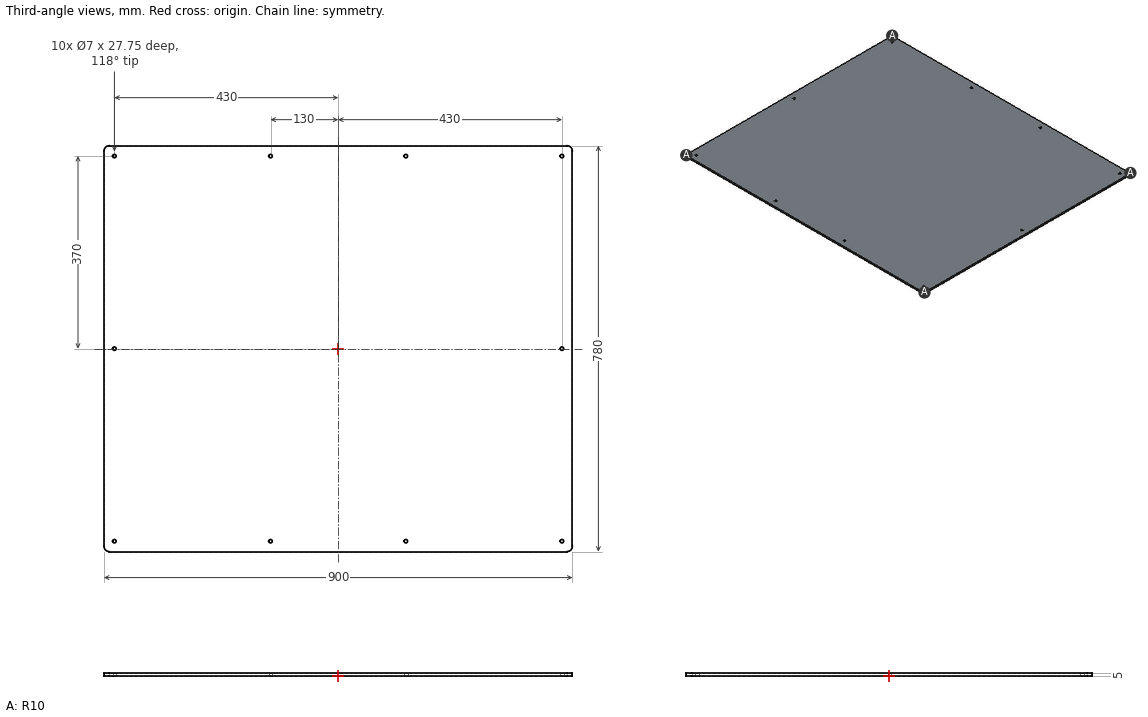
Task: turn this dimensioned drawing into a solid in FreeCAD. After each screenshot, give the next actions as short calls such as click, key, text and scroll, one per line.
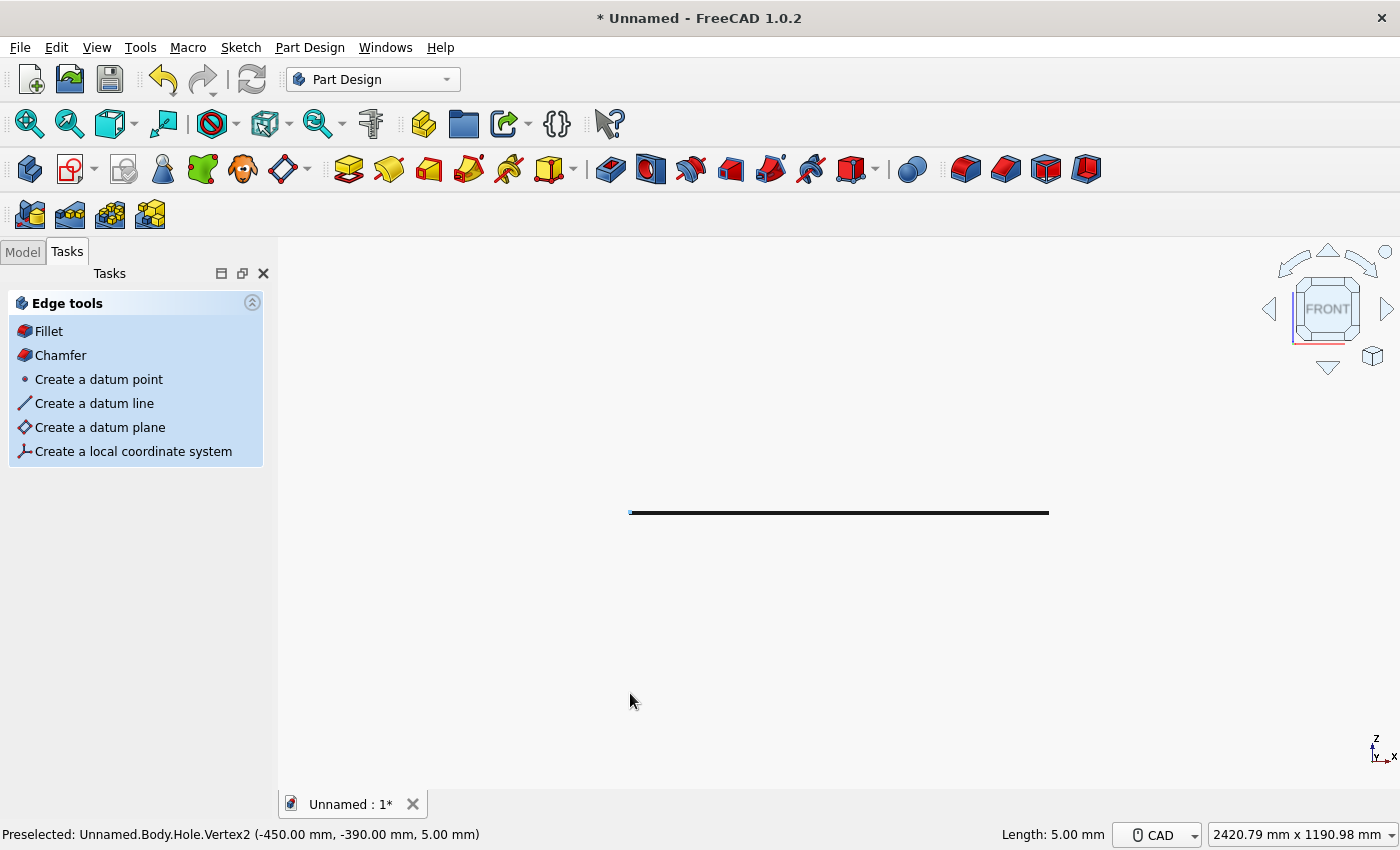
scroll(630, 512, up, 15)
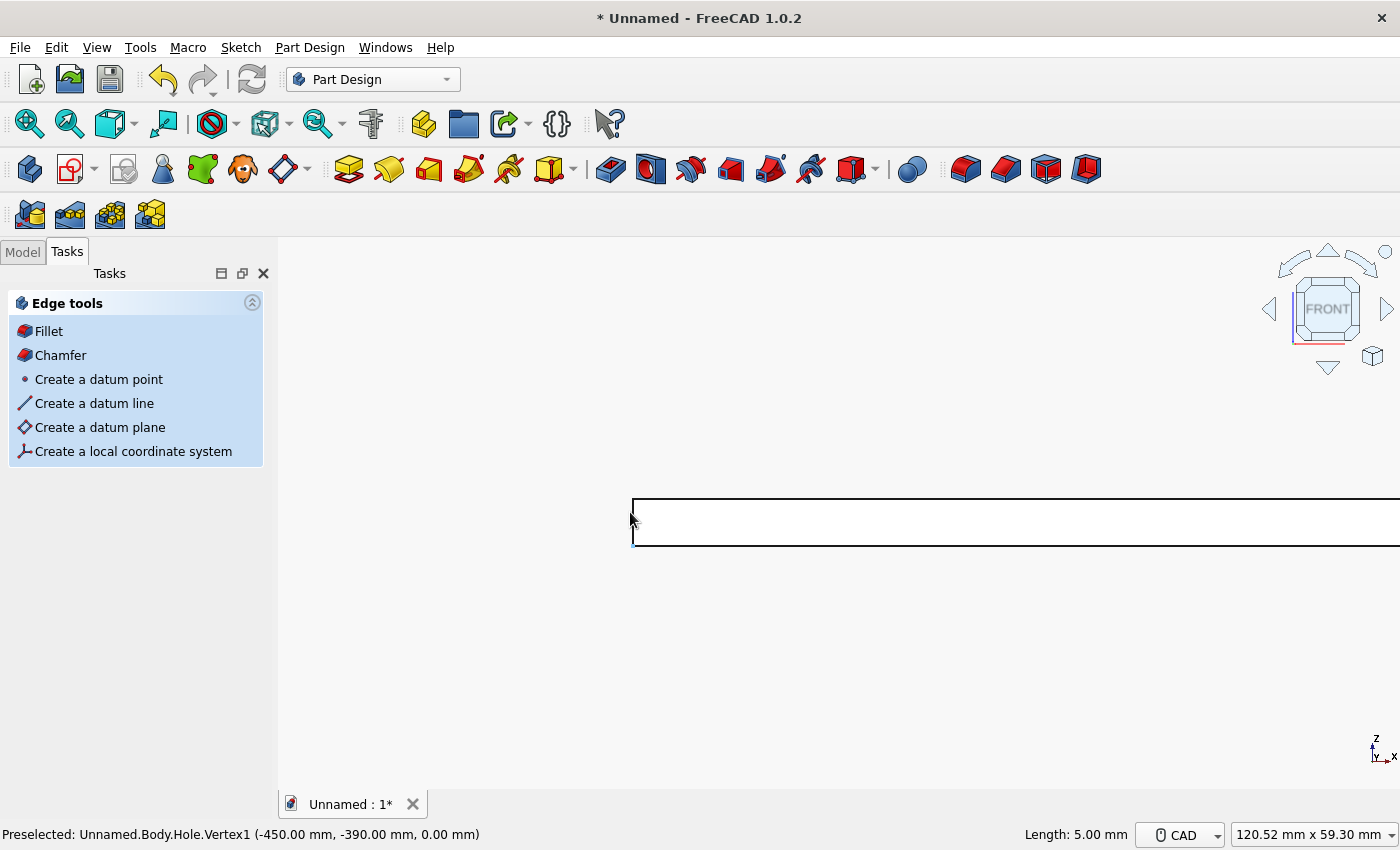
click(633, 522, ctrl)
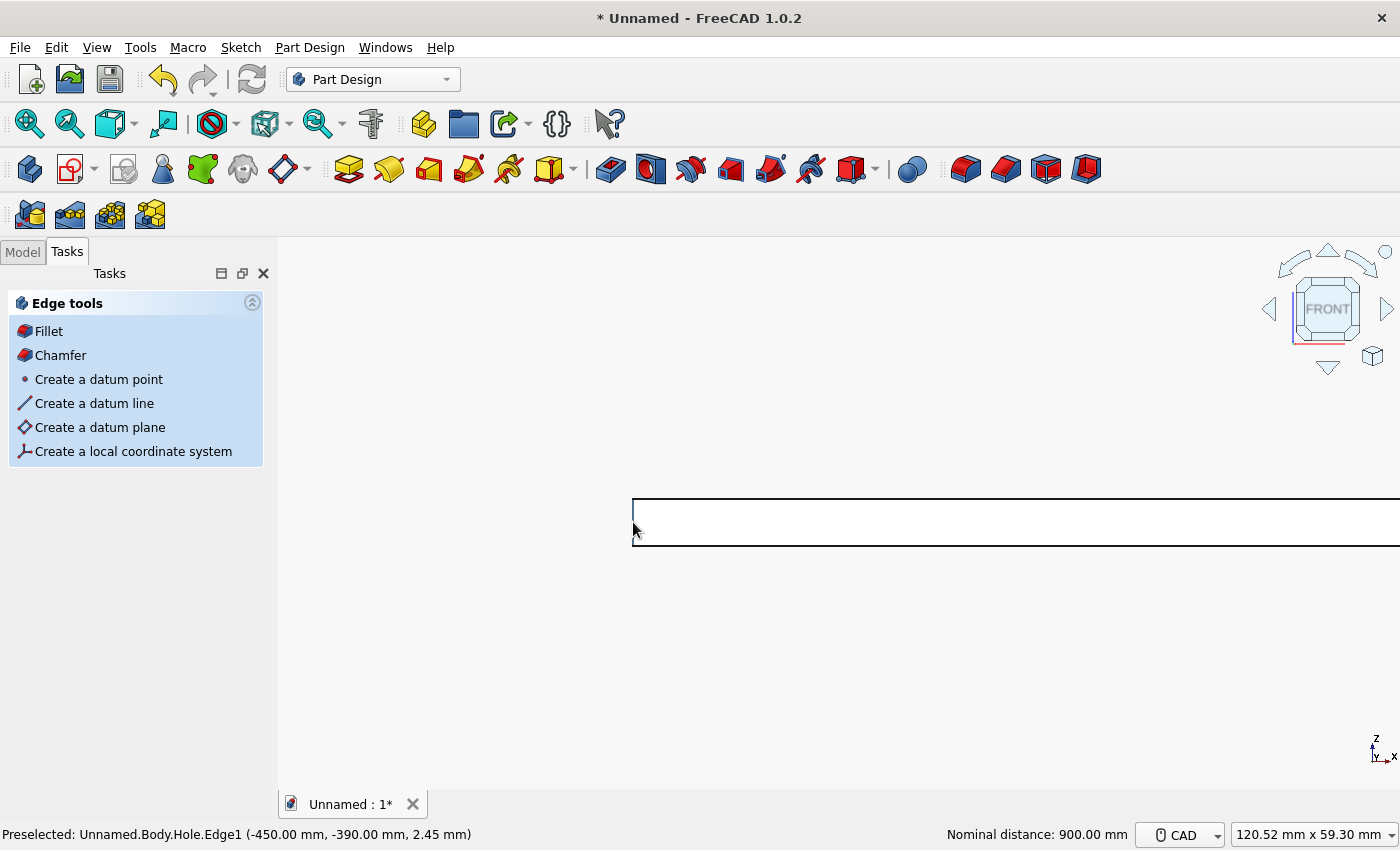
click(30, 124)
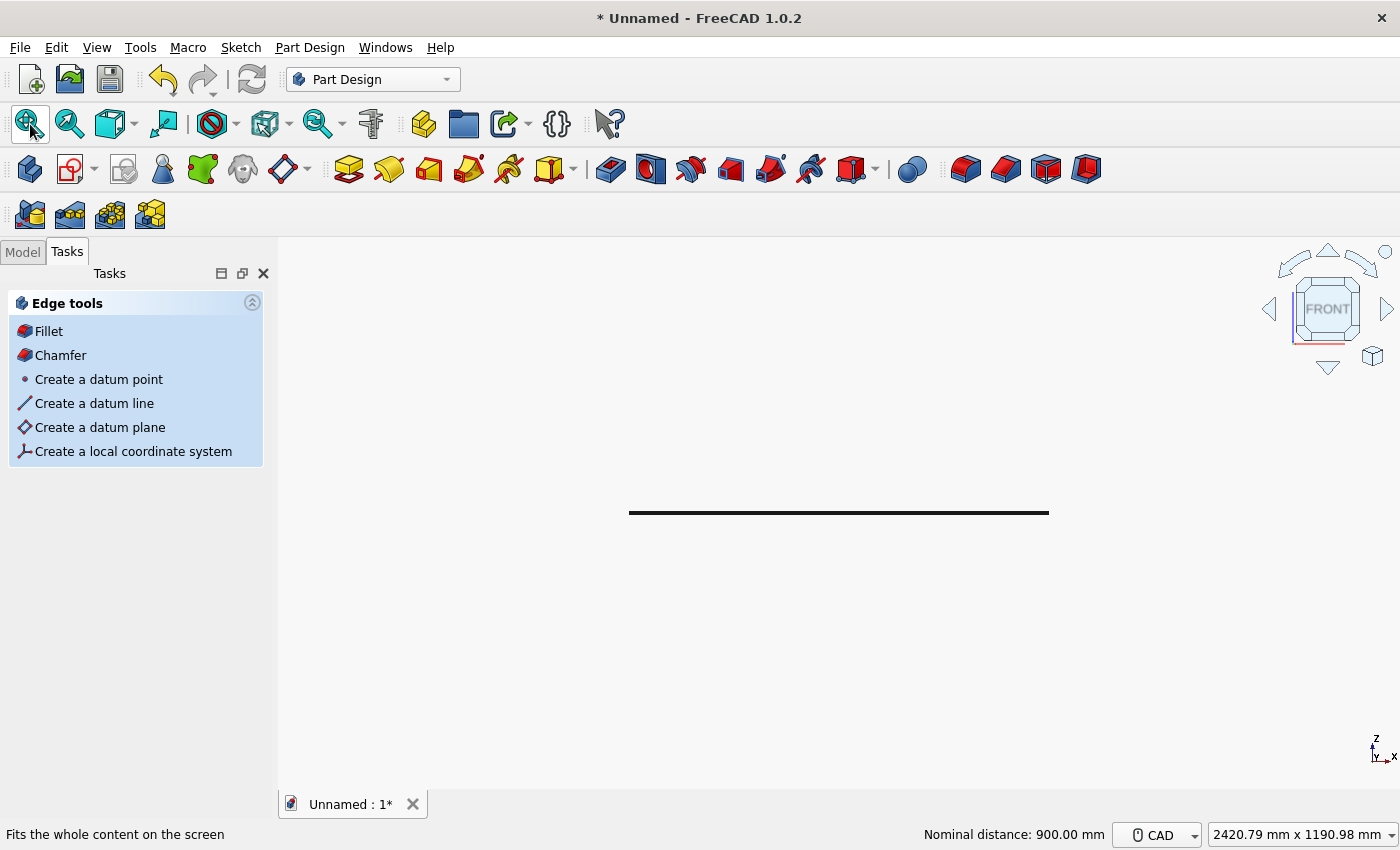
key(3)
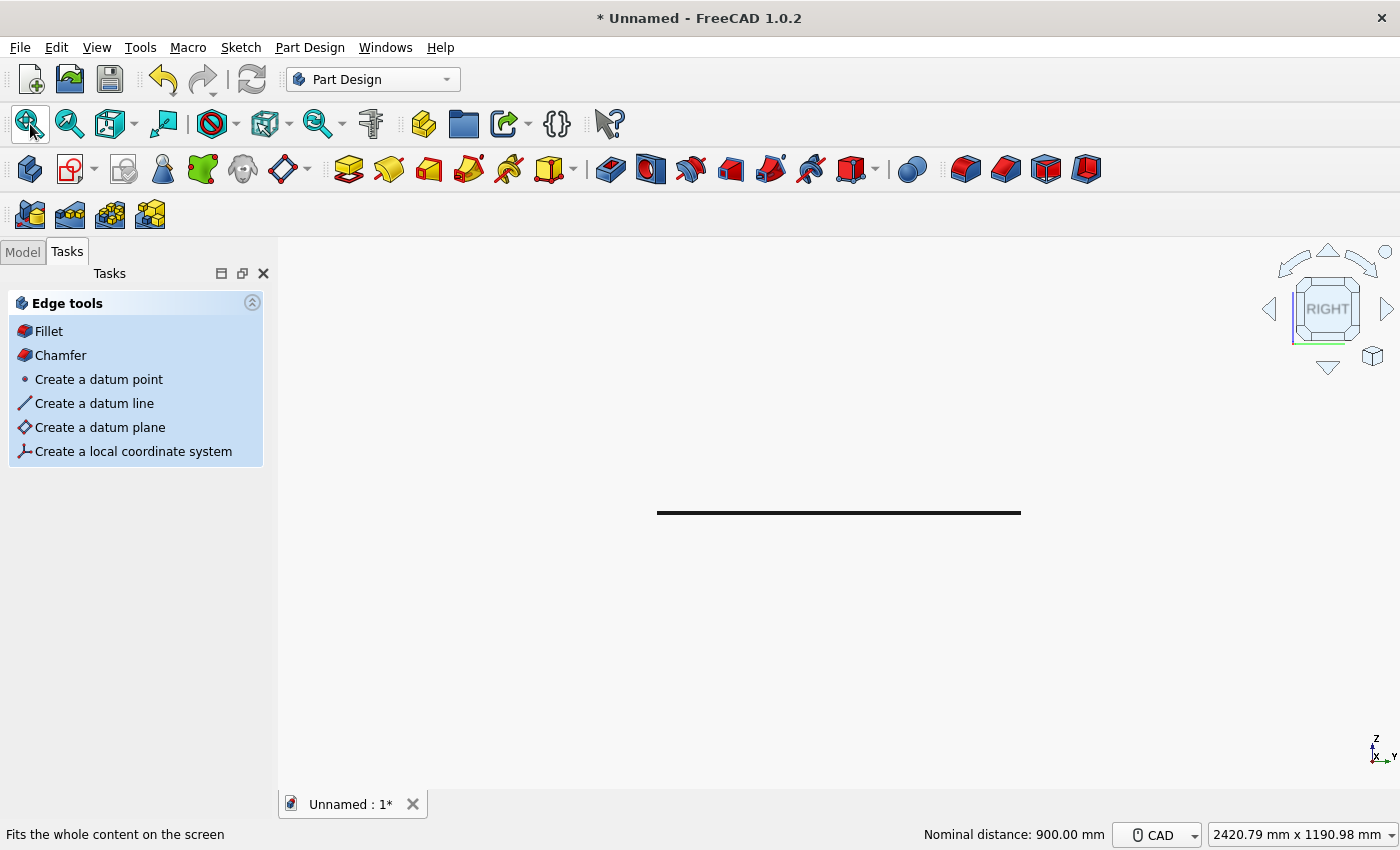
click(30, 124)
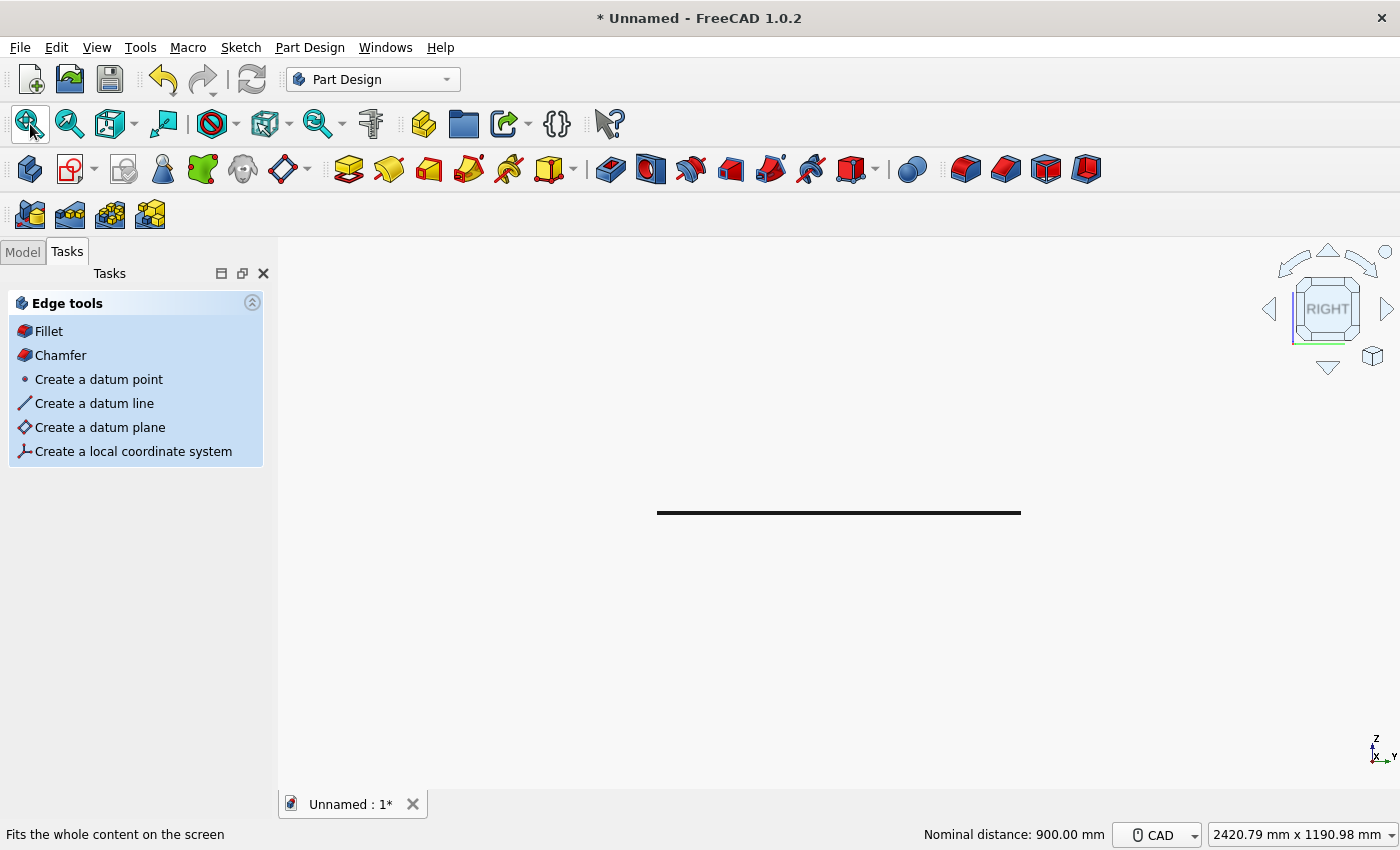
scroll(1020, 512, up, 15)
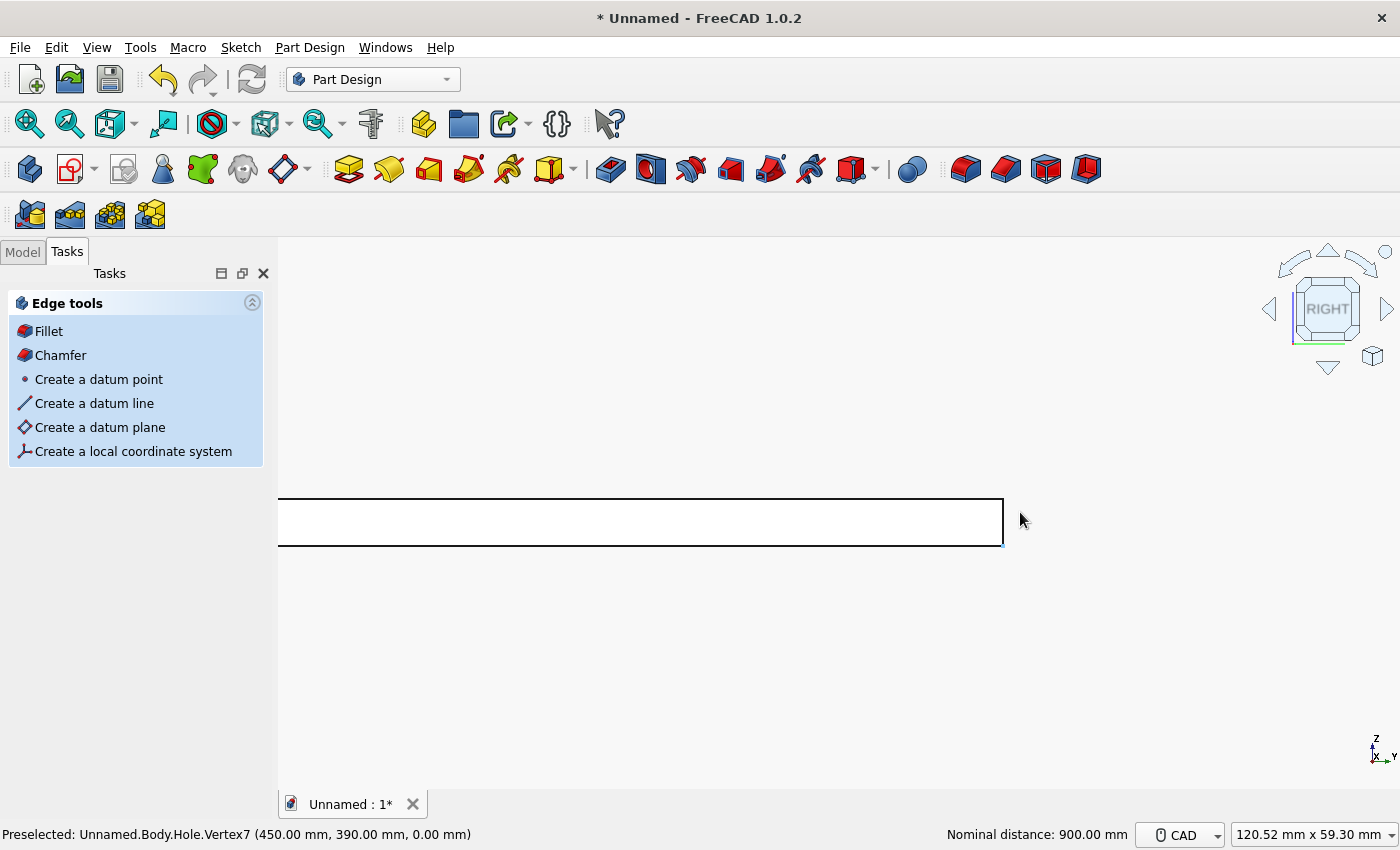
click(1003, 522, ctrl)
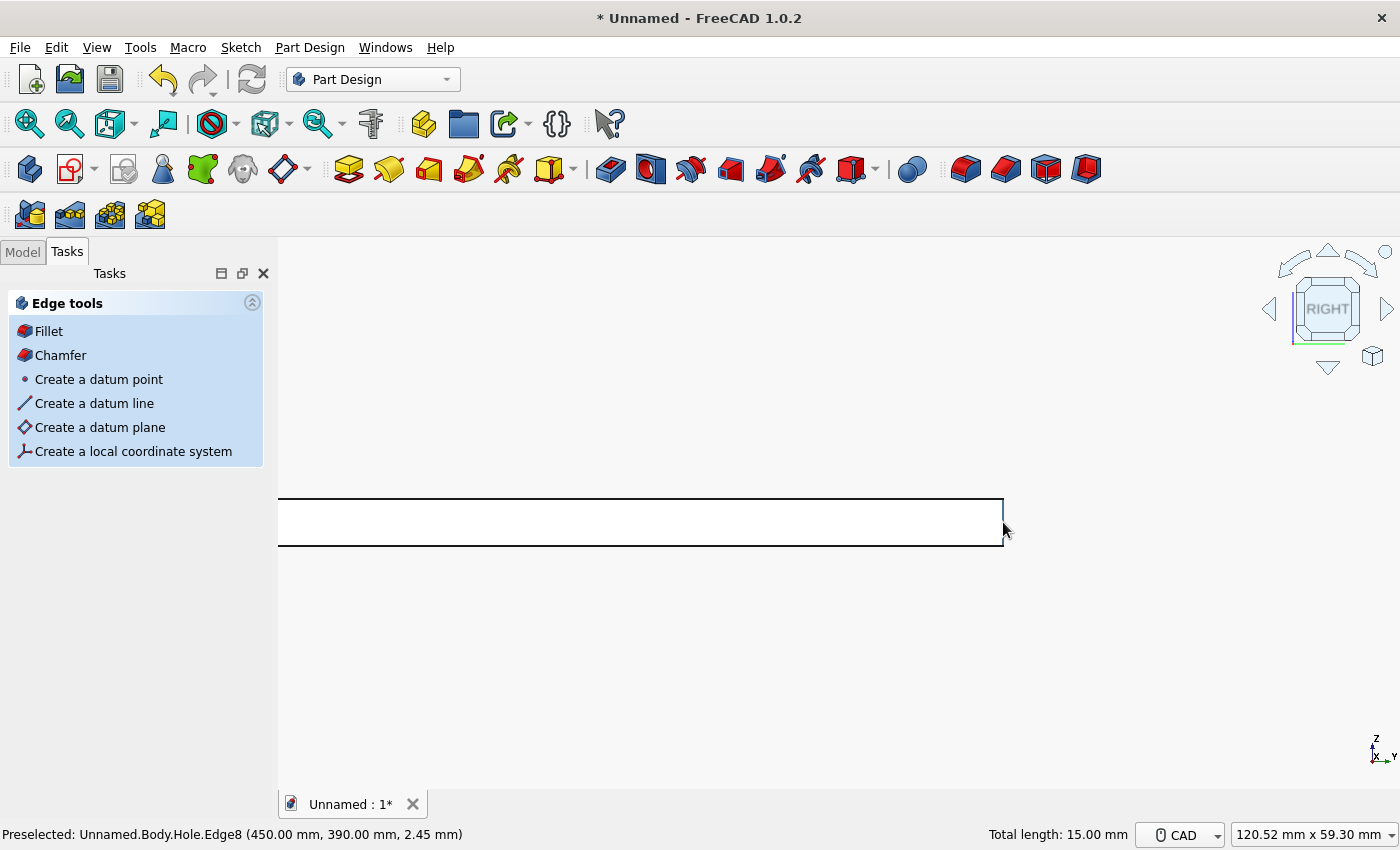
click(30, 124)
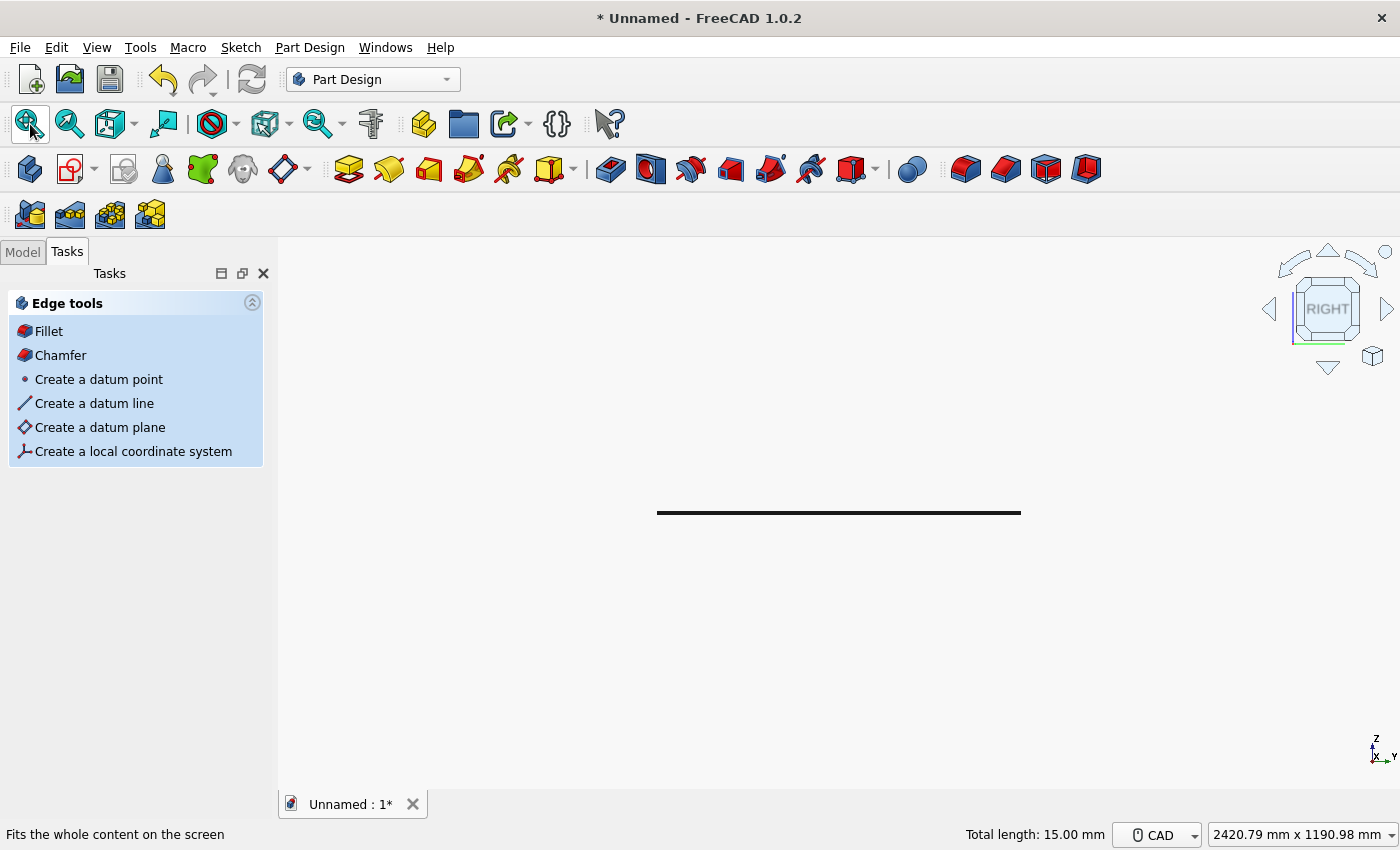
key(5)